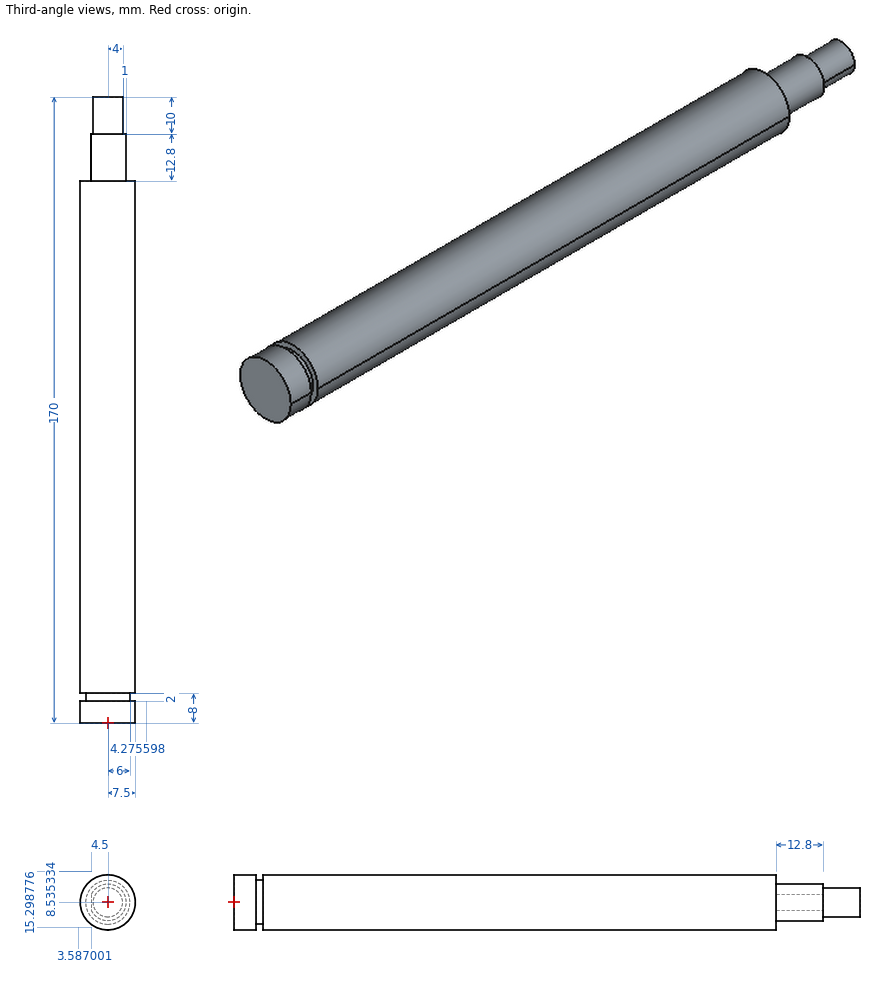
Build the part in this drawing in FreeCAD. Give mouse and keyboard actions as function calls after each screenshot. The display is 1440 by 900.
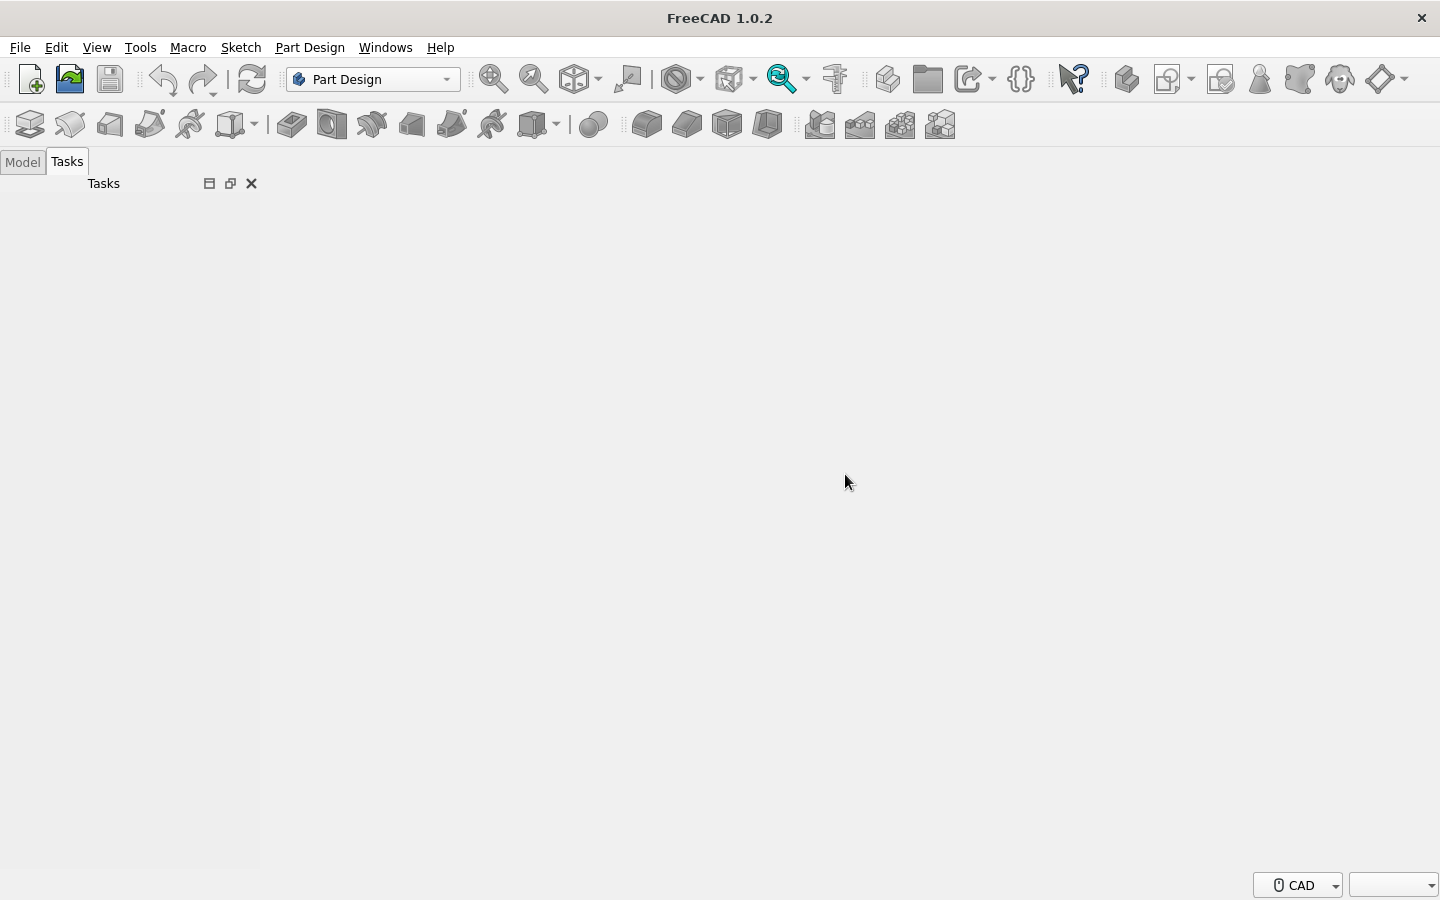
click(30, 80)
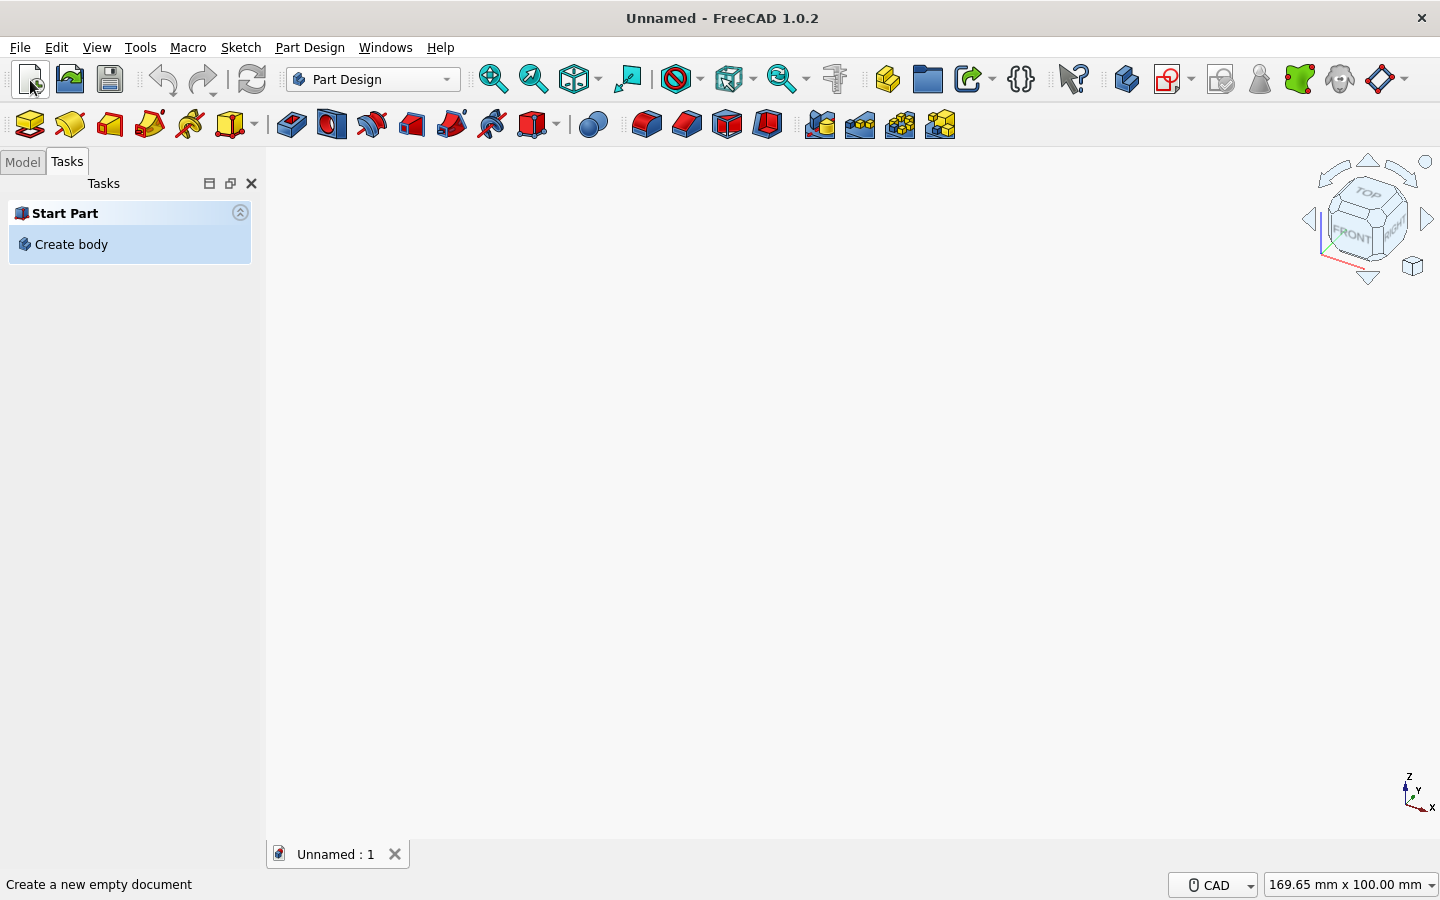
click(1168, 80)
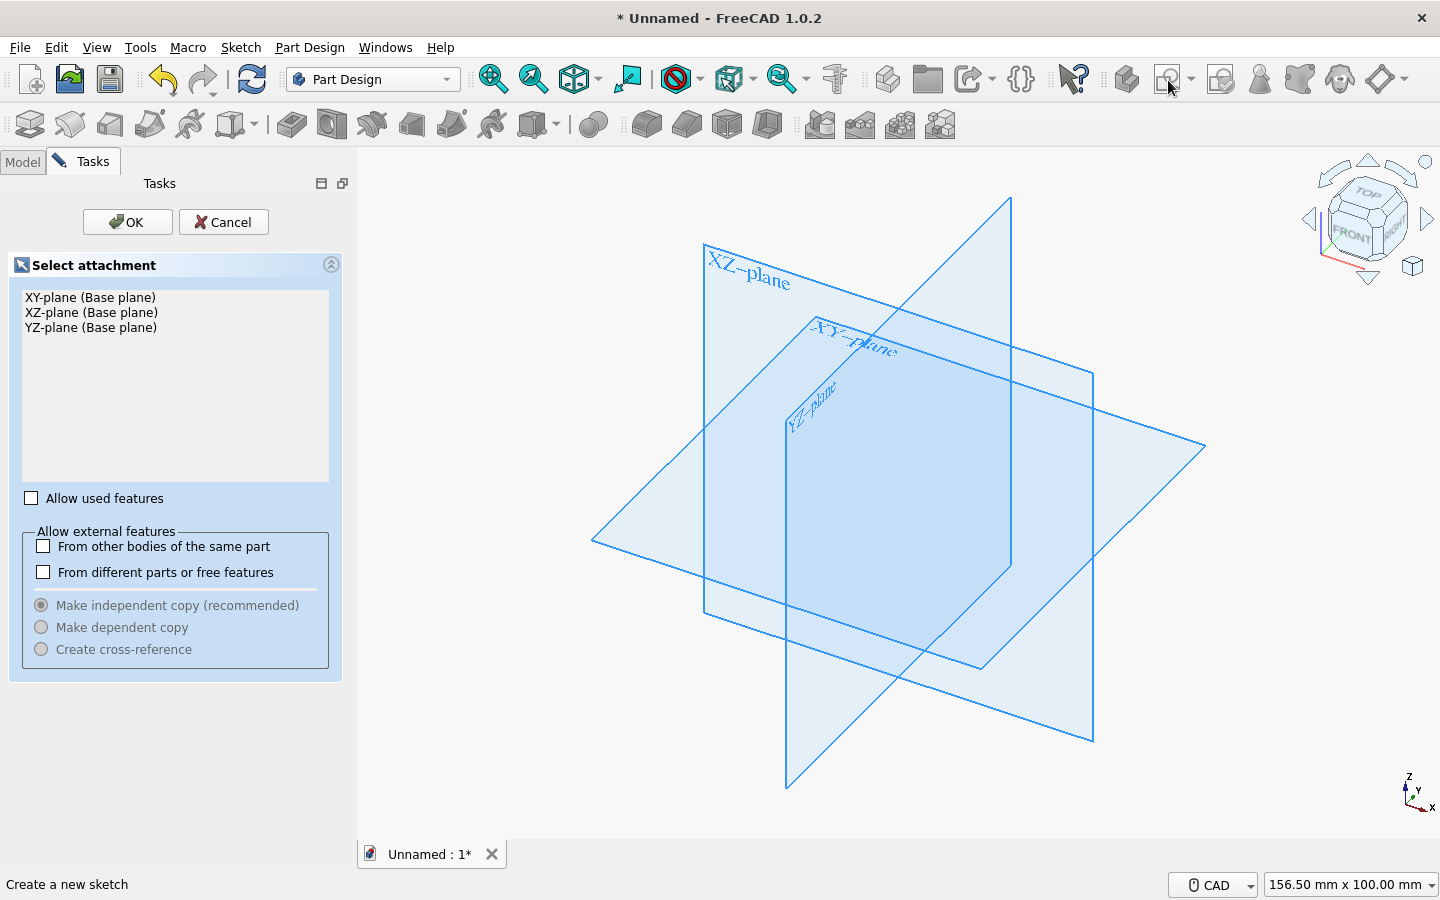
click(82, 298)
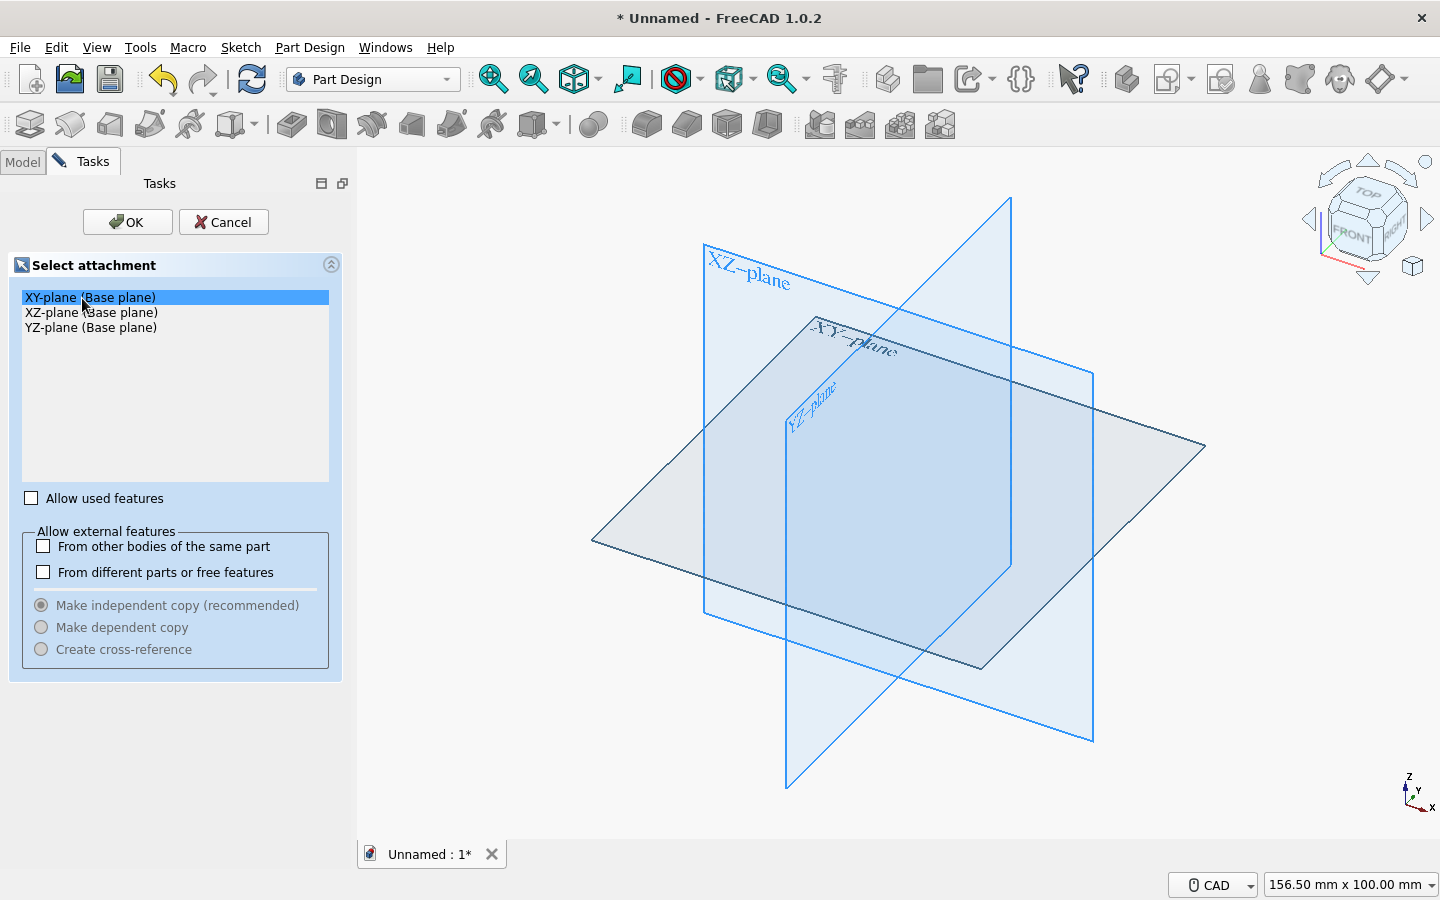
click(128, 222)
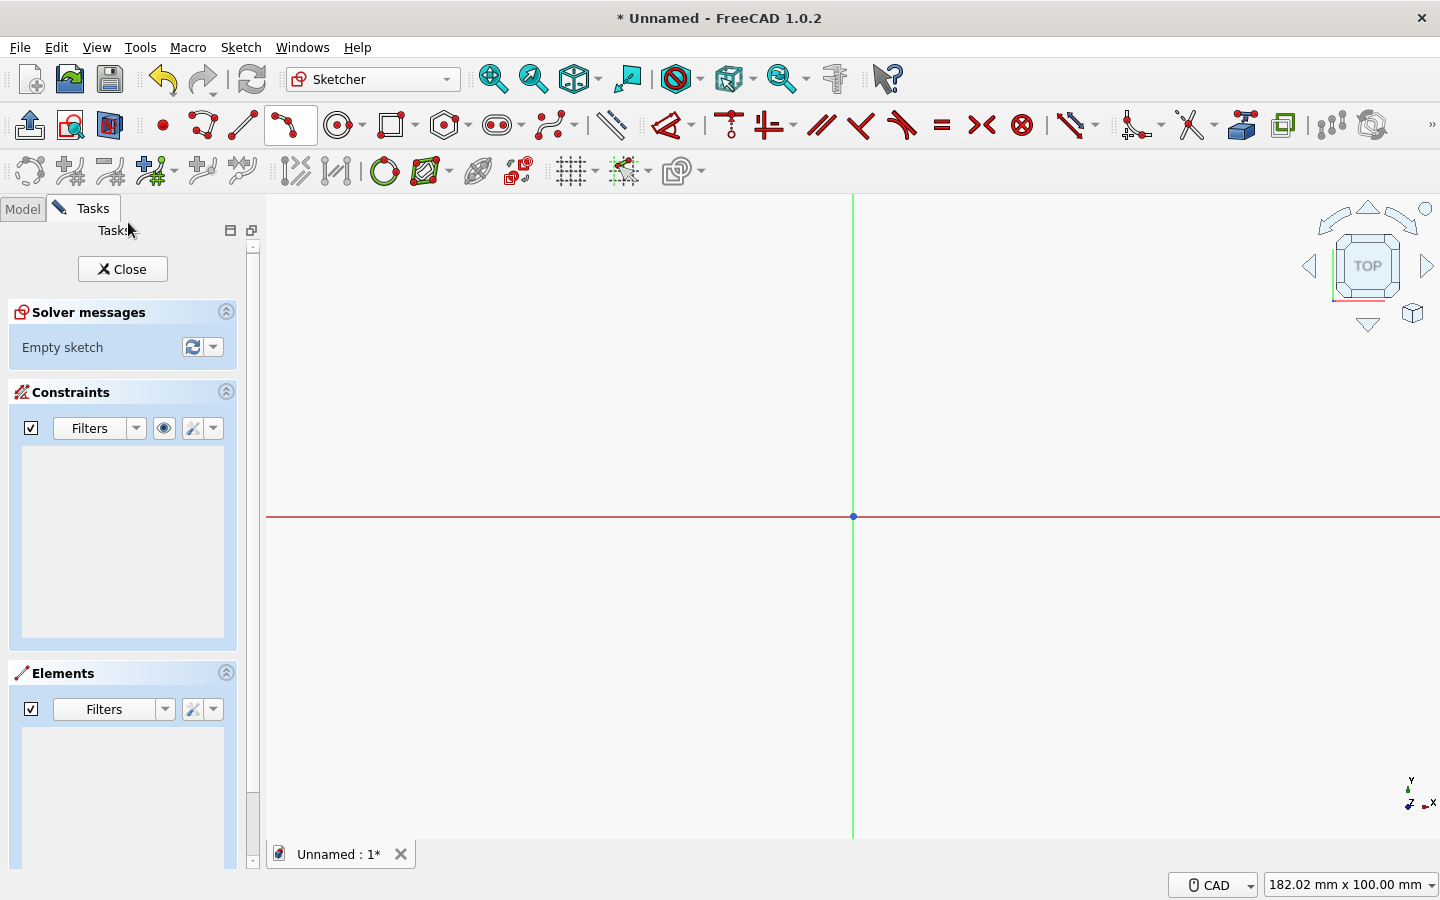
scroll(731, 811, down, 5)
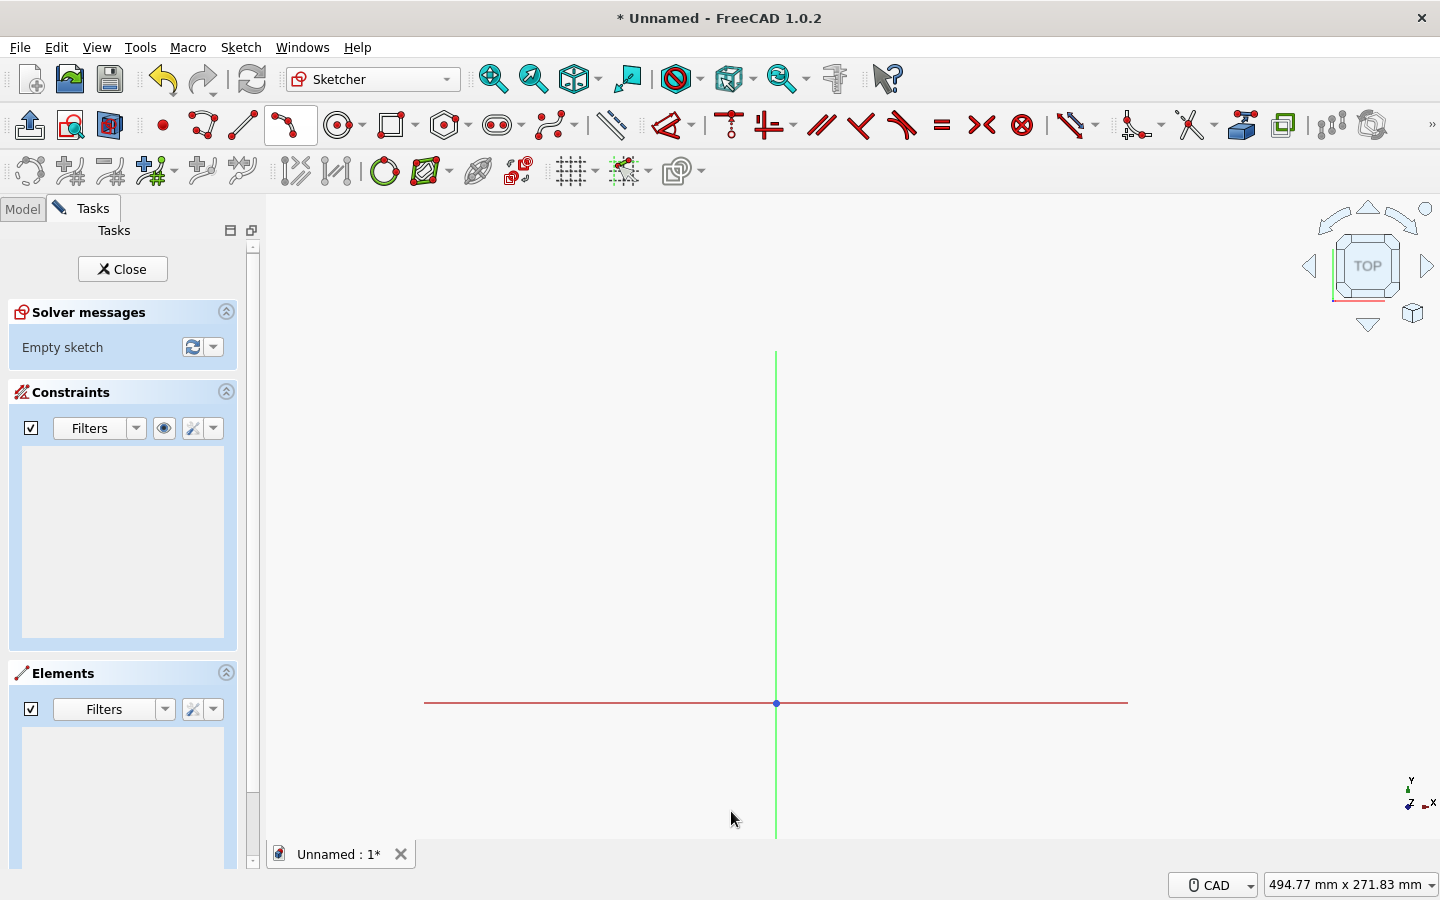
click(204, 126)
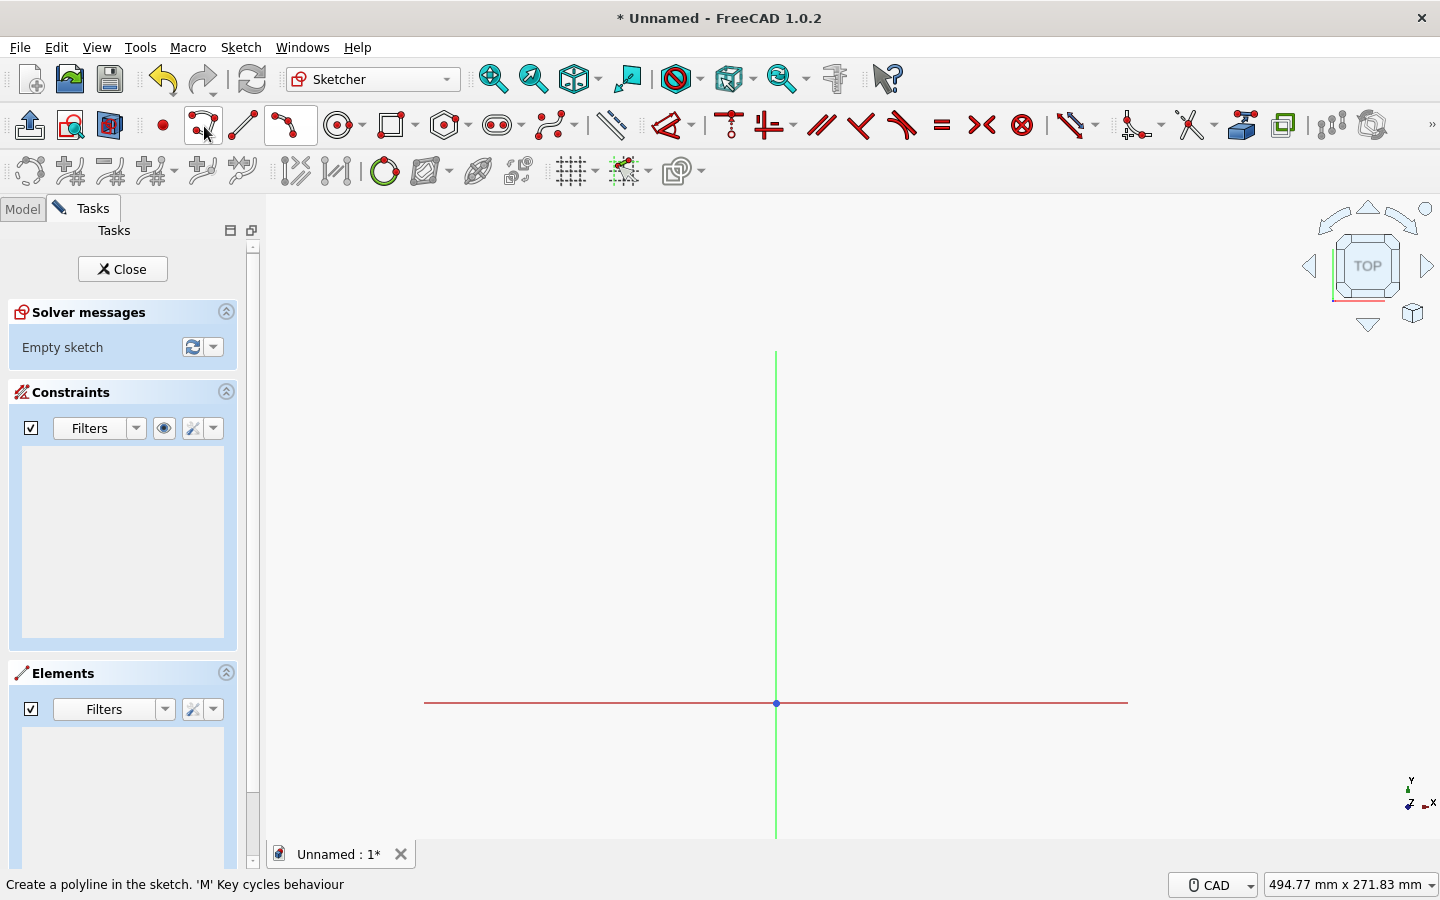
click(776, 703)
click(794, 694)
click(794, 354)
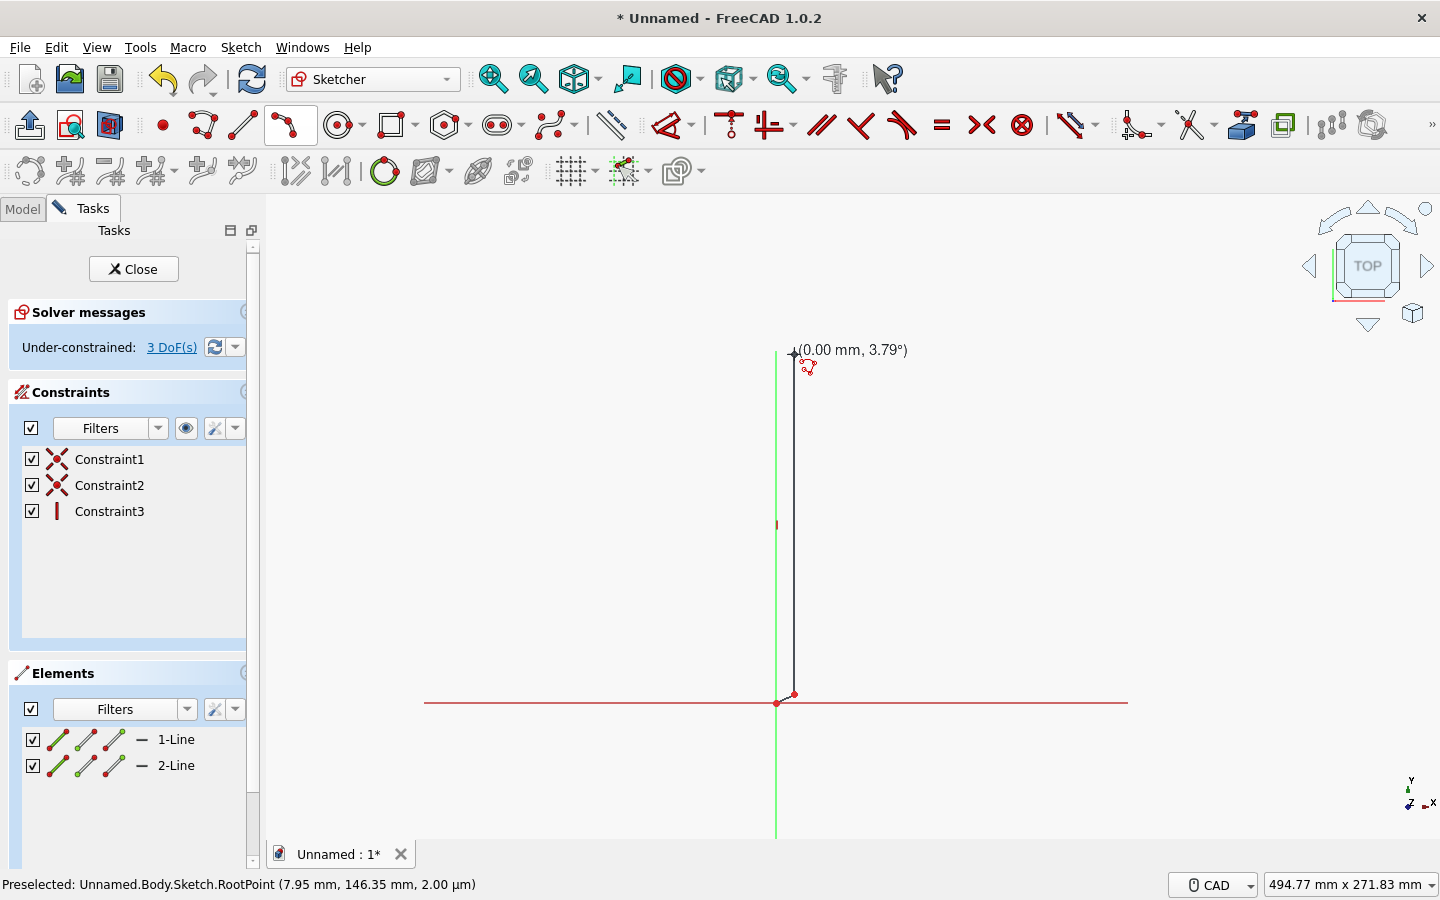
scroll(788, 354, up, 5)